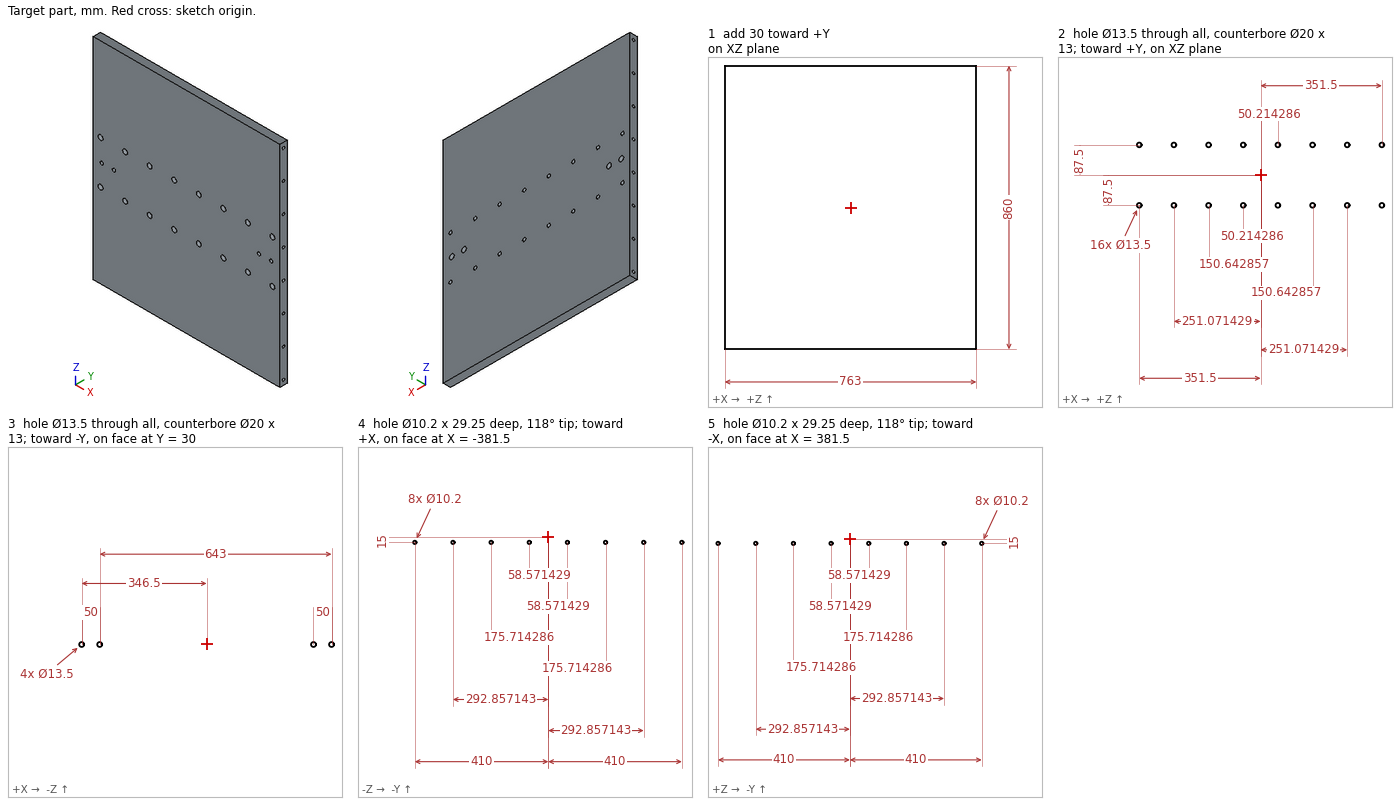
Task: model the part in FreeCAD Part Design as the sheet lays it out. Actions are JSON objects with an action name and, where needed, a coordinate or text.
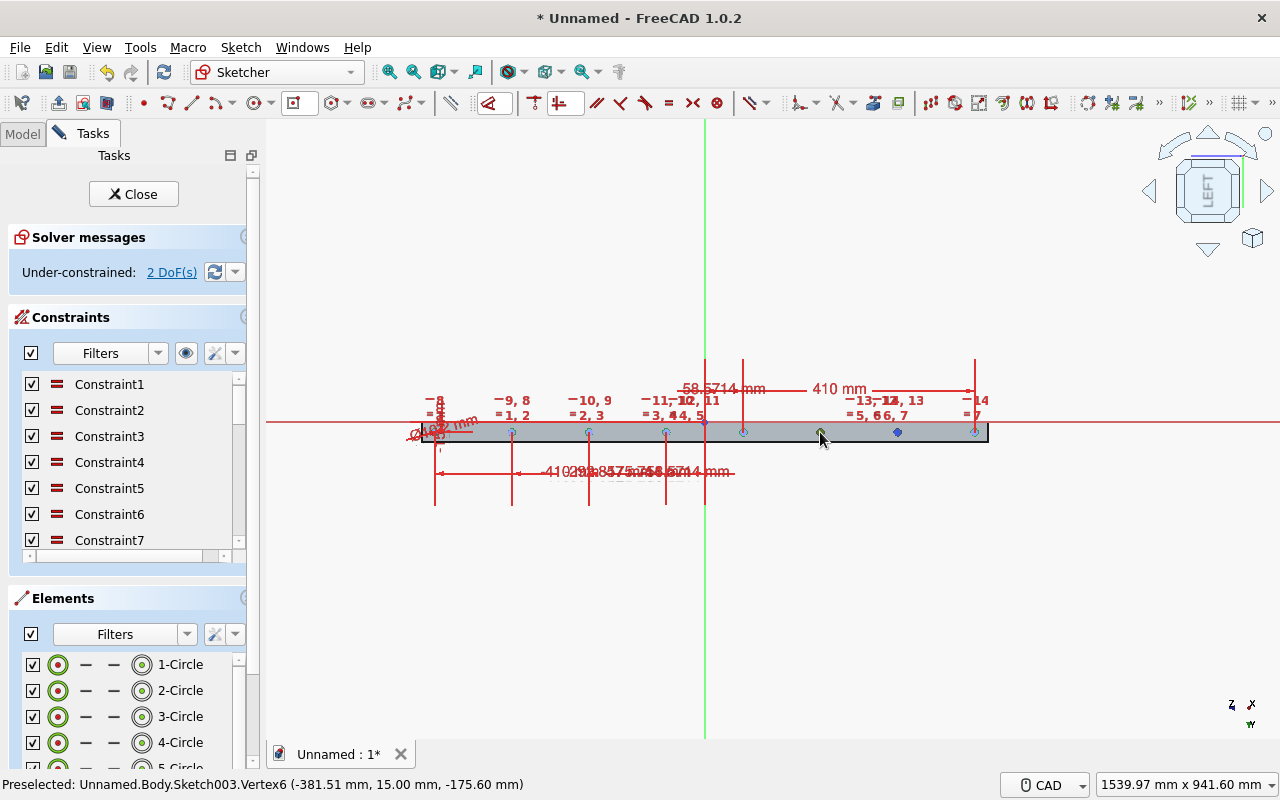
{"action": "key", "text": "l"}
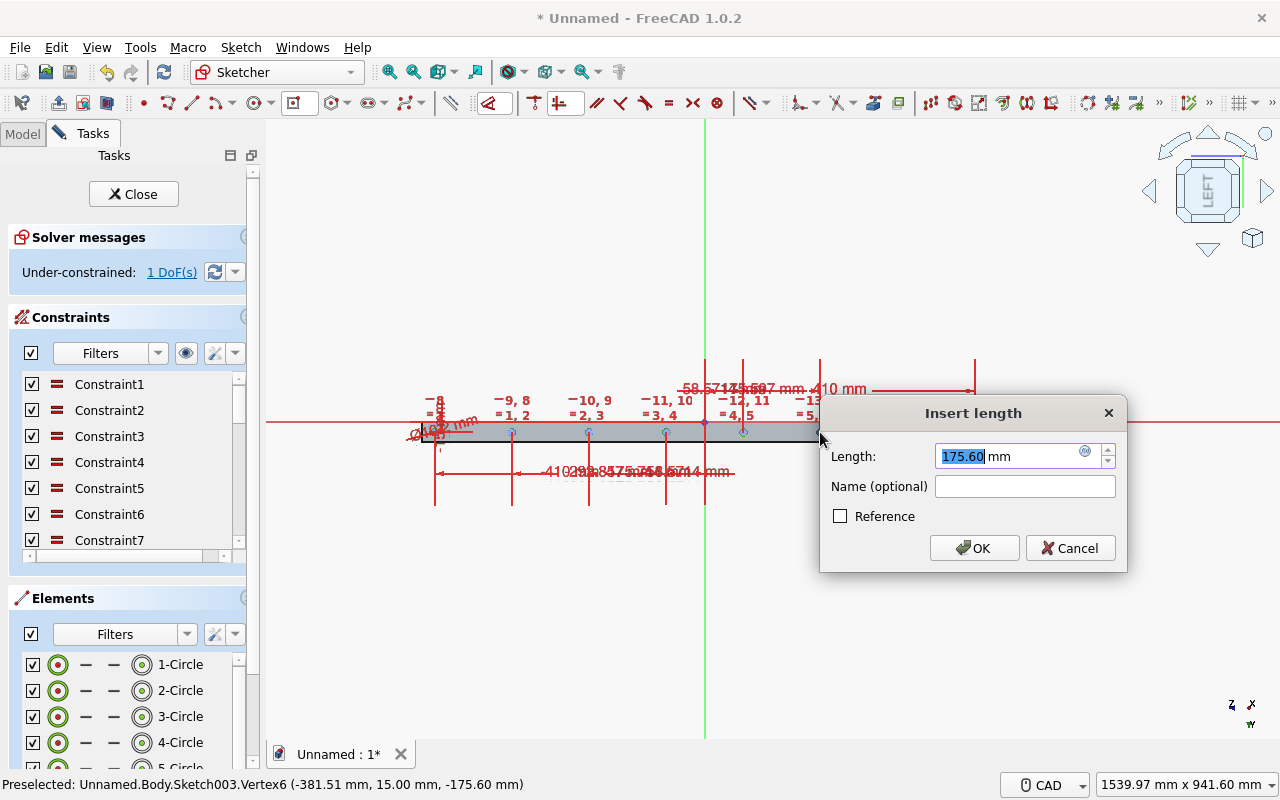
{"action": "type", "text": "175.714286"}
{"action": "key", "text": "Return"}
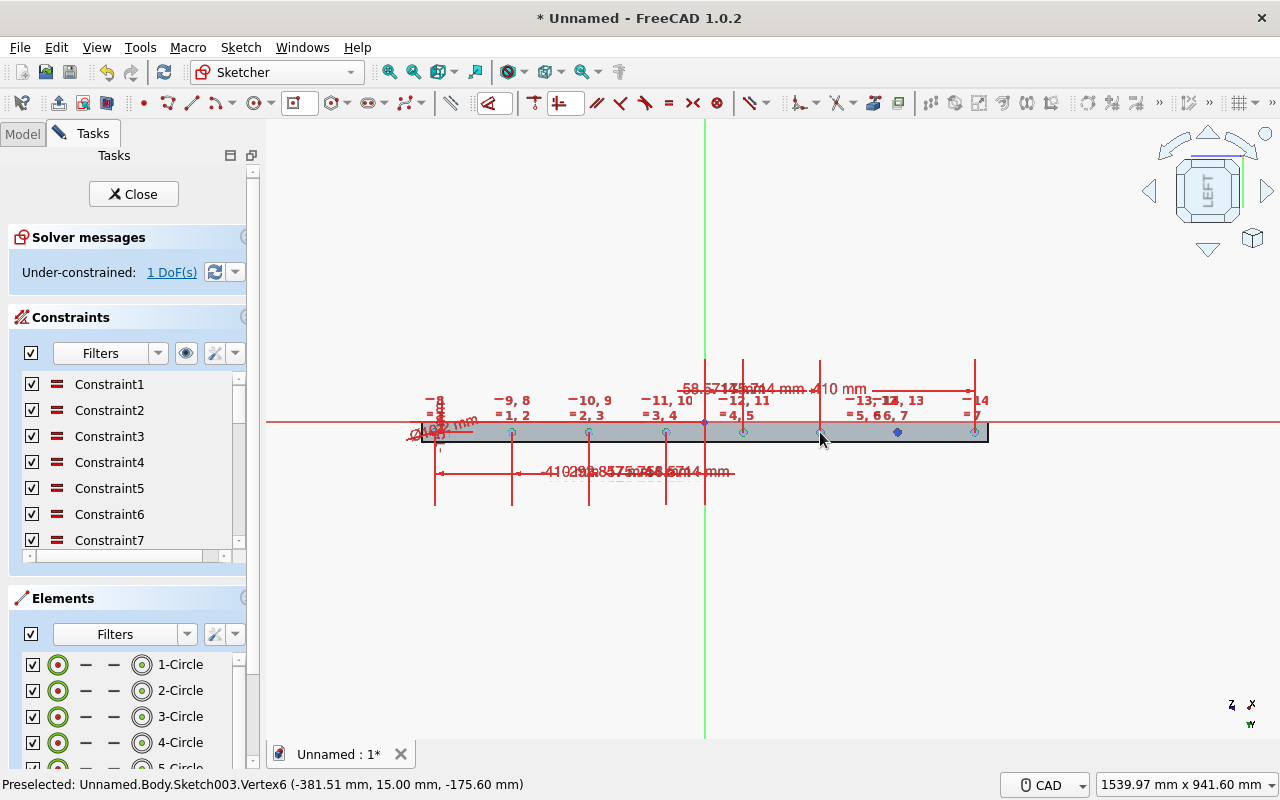
{"action": "left_click", "coordinate": [898, 432]}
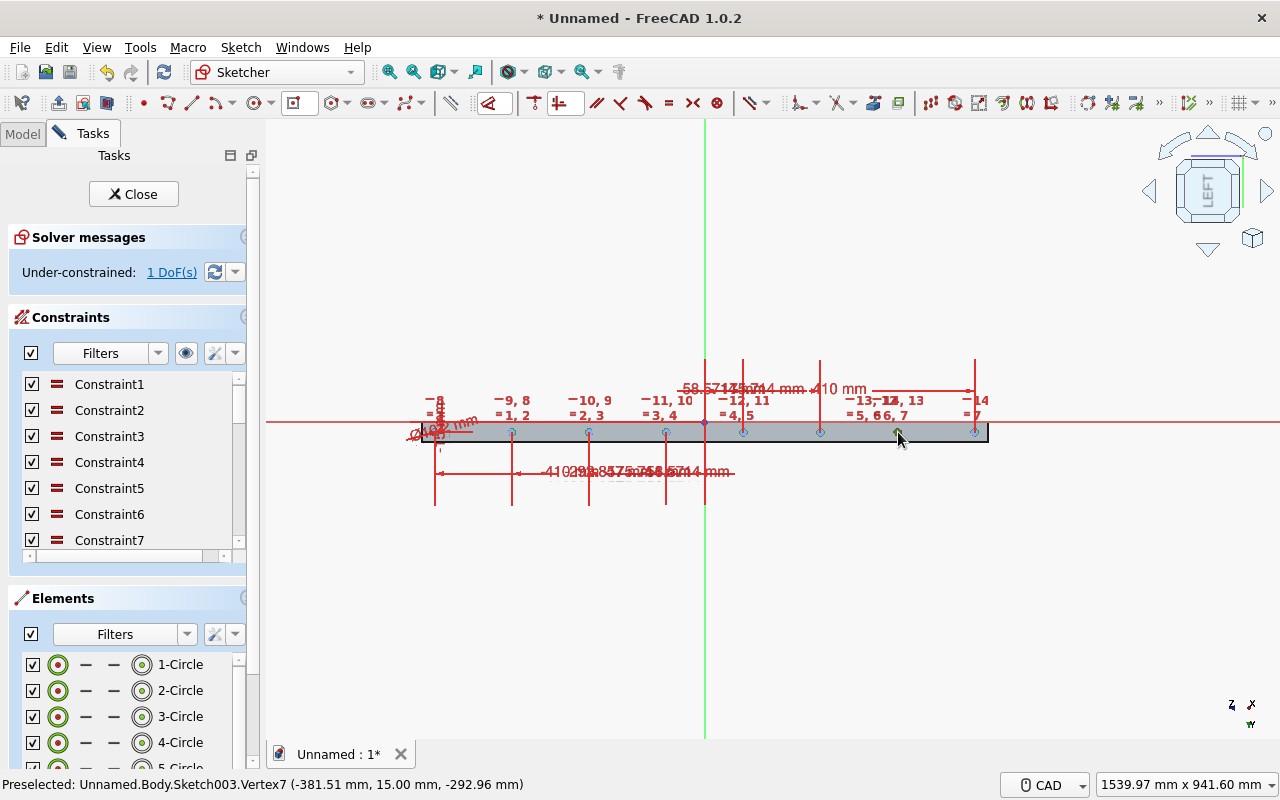
{"action": "key", "text": "l"}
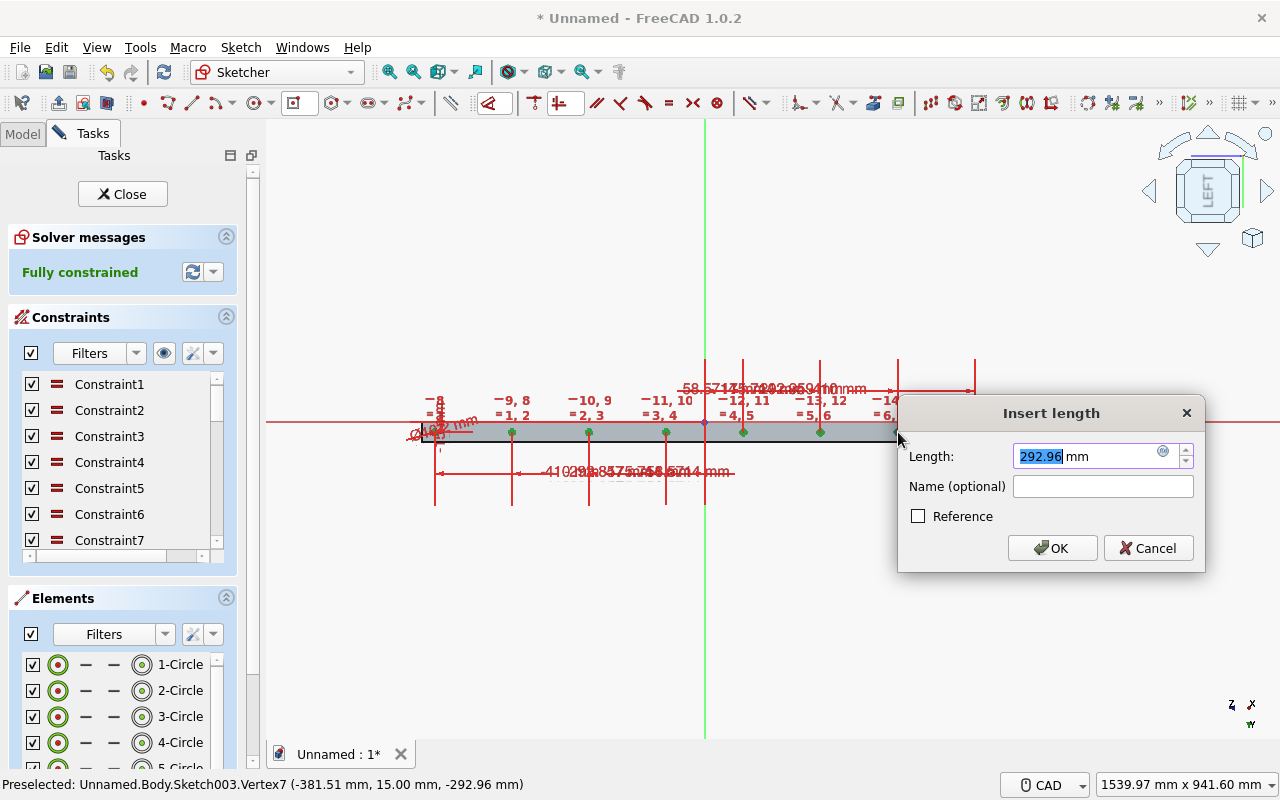
{"action": "type", "text": "292.857143"}
{"action": "key", "text": "Return"}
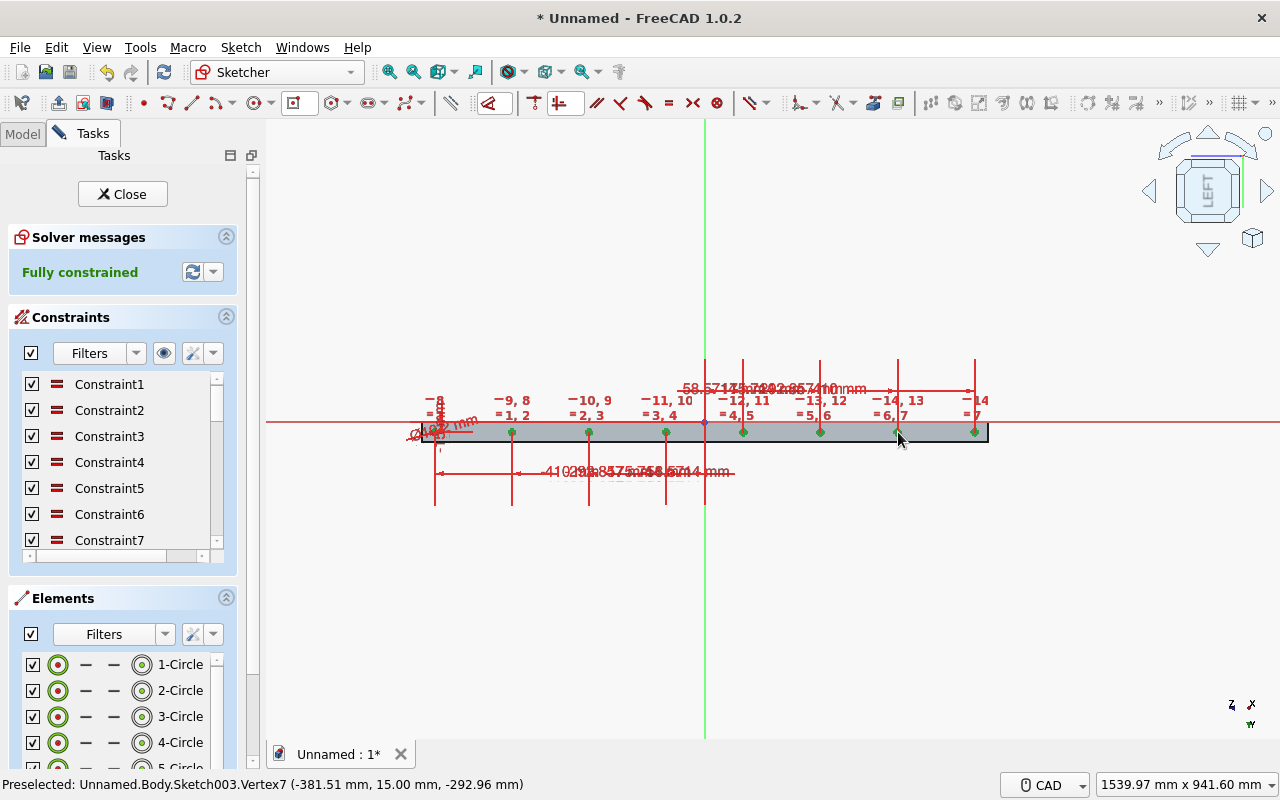
{"action": "left_click", "coordinate": [123, 194]}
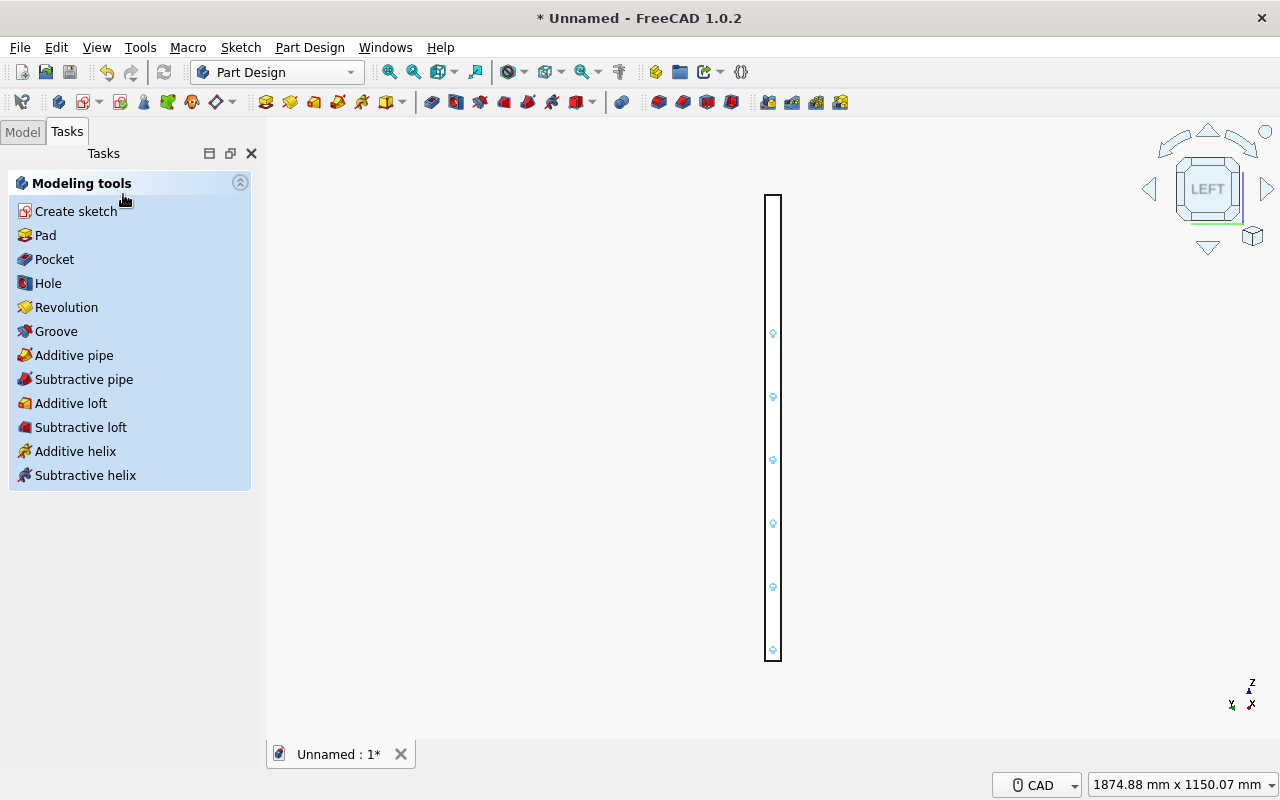
{"action": "left_click", "coordinate": [456, 102]}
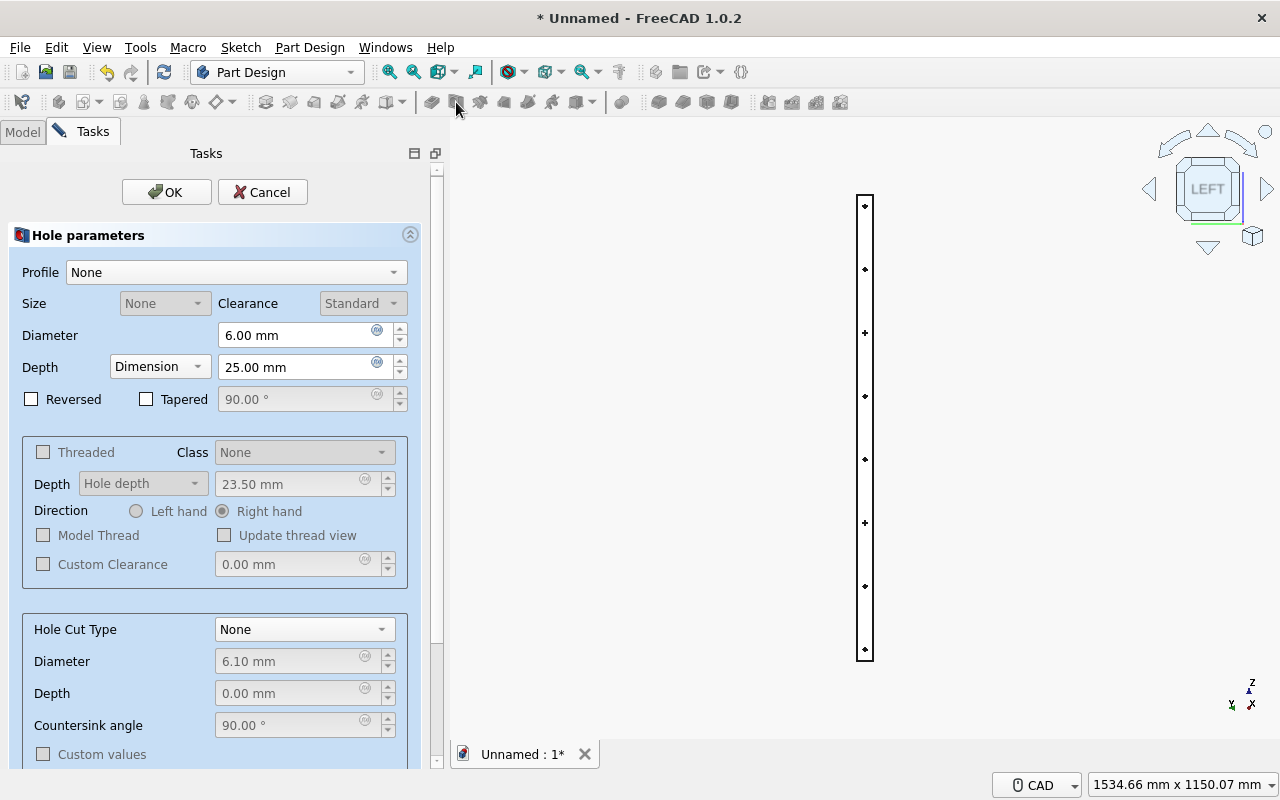
{"action": "triple_click", "coordinate": [305, 335]}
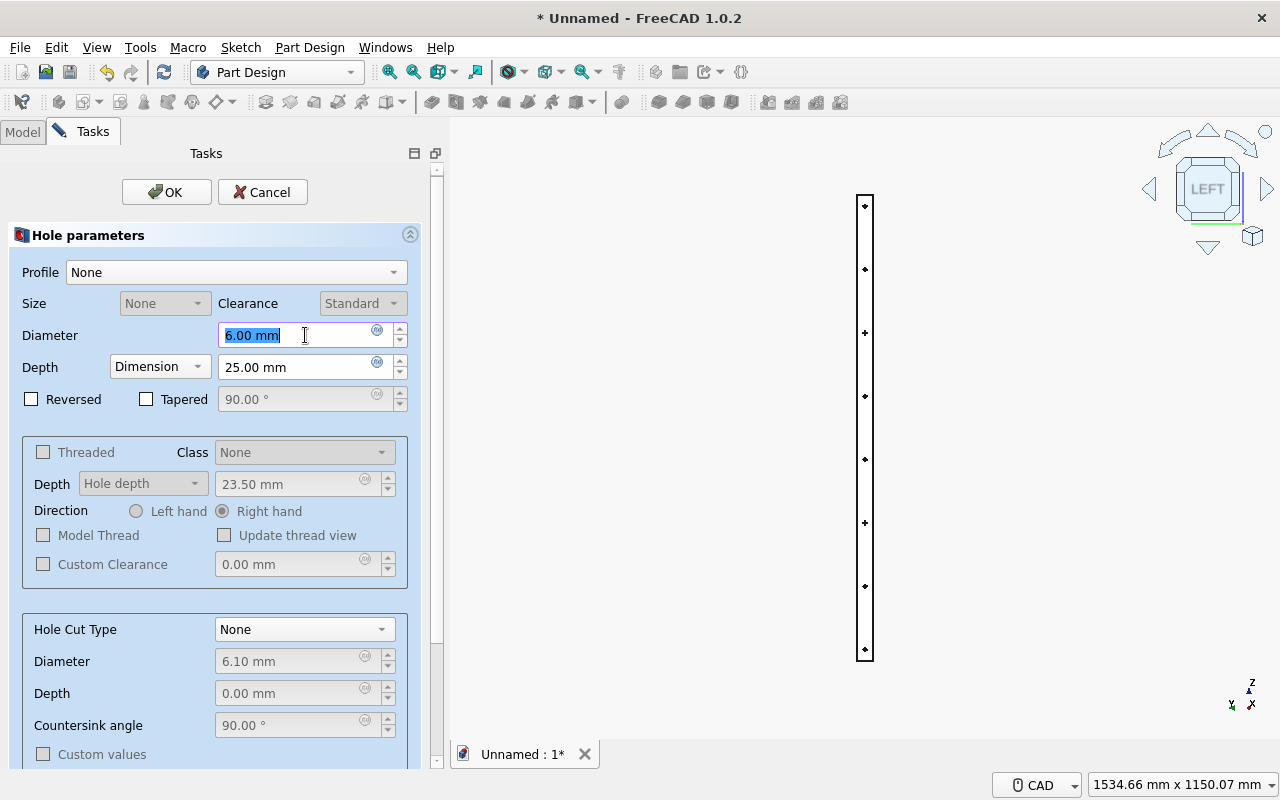
{"action": "type", "text": "10.2"}
{"action": "key", "text": "Tab"}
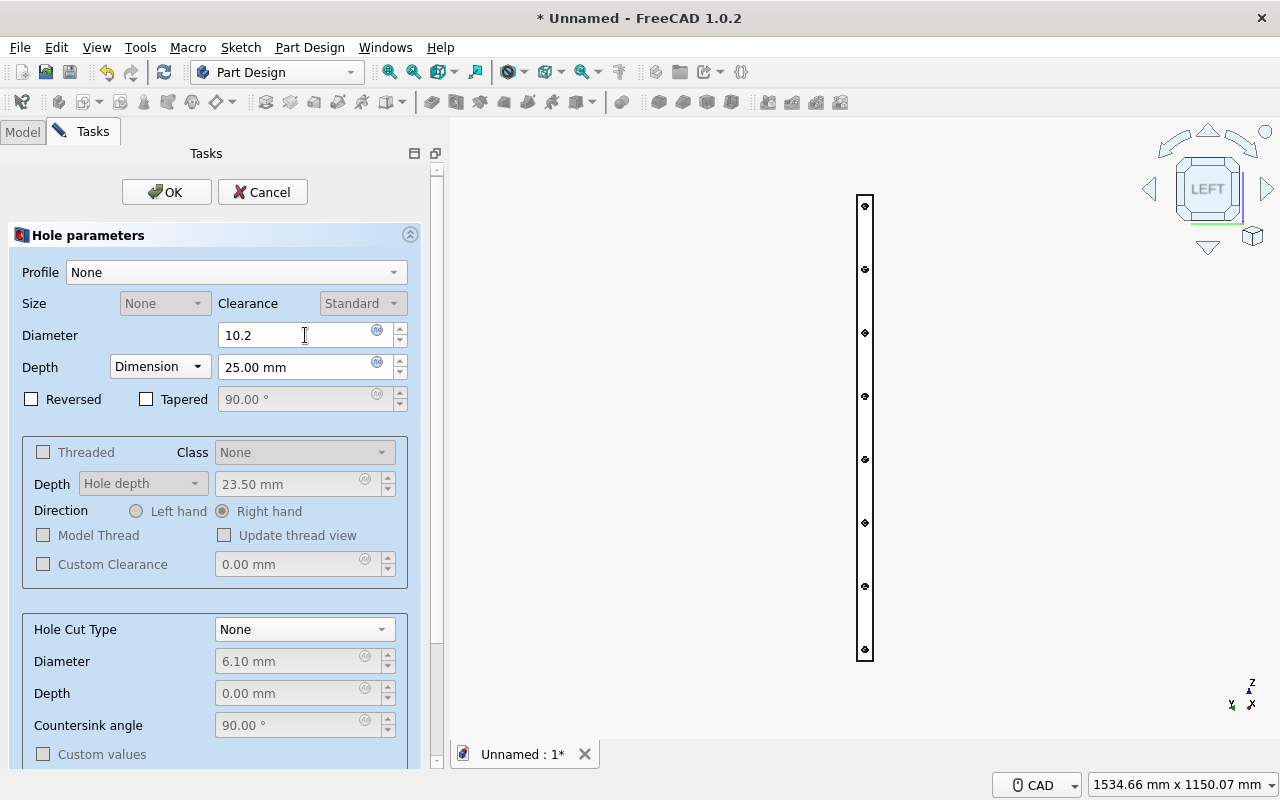
{"action": "triple_click", "coordinate": [305, 367]}